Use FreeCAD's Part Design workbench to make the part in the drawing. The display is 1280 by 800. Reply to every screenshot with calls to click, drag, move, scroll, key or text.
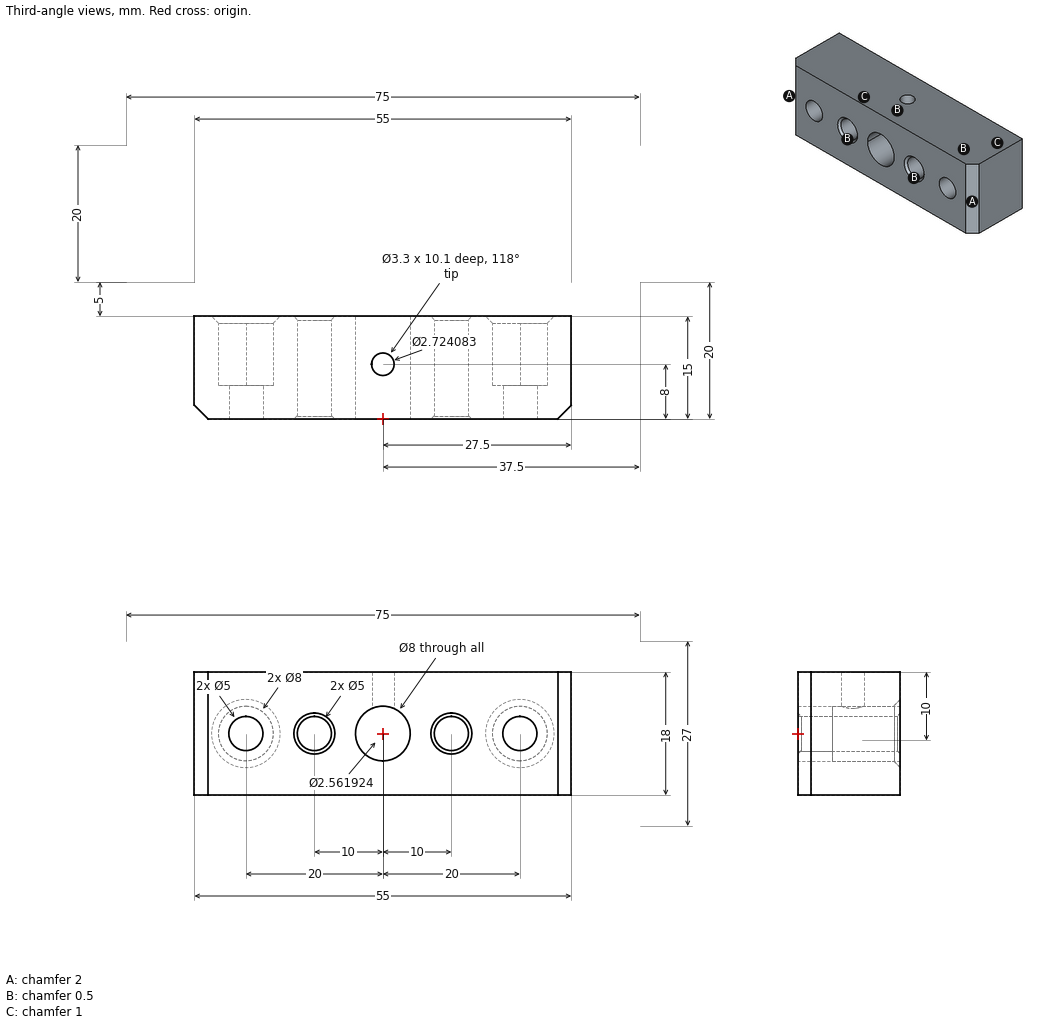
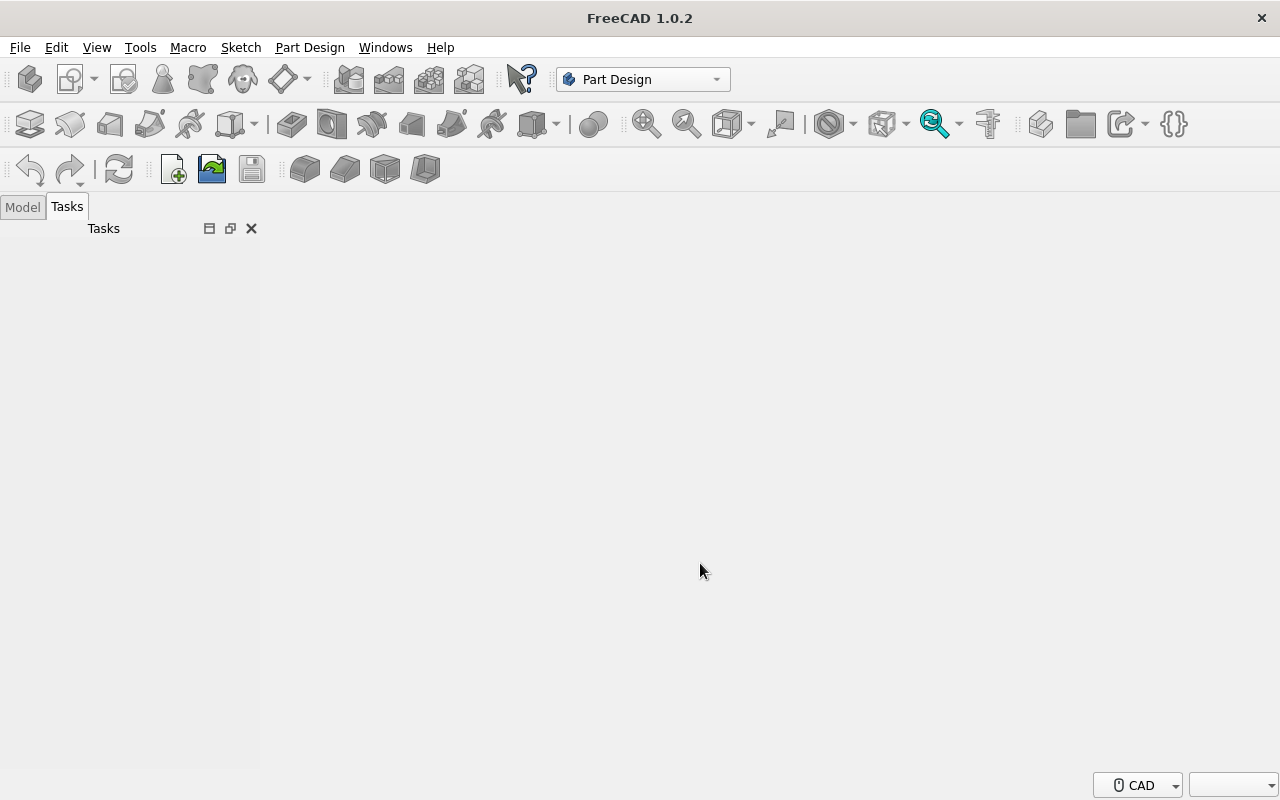
click(172, 170)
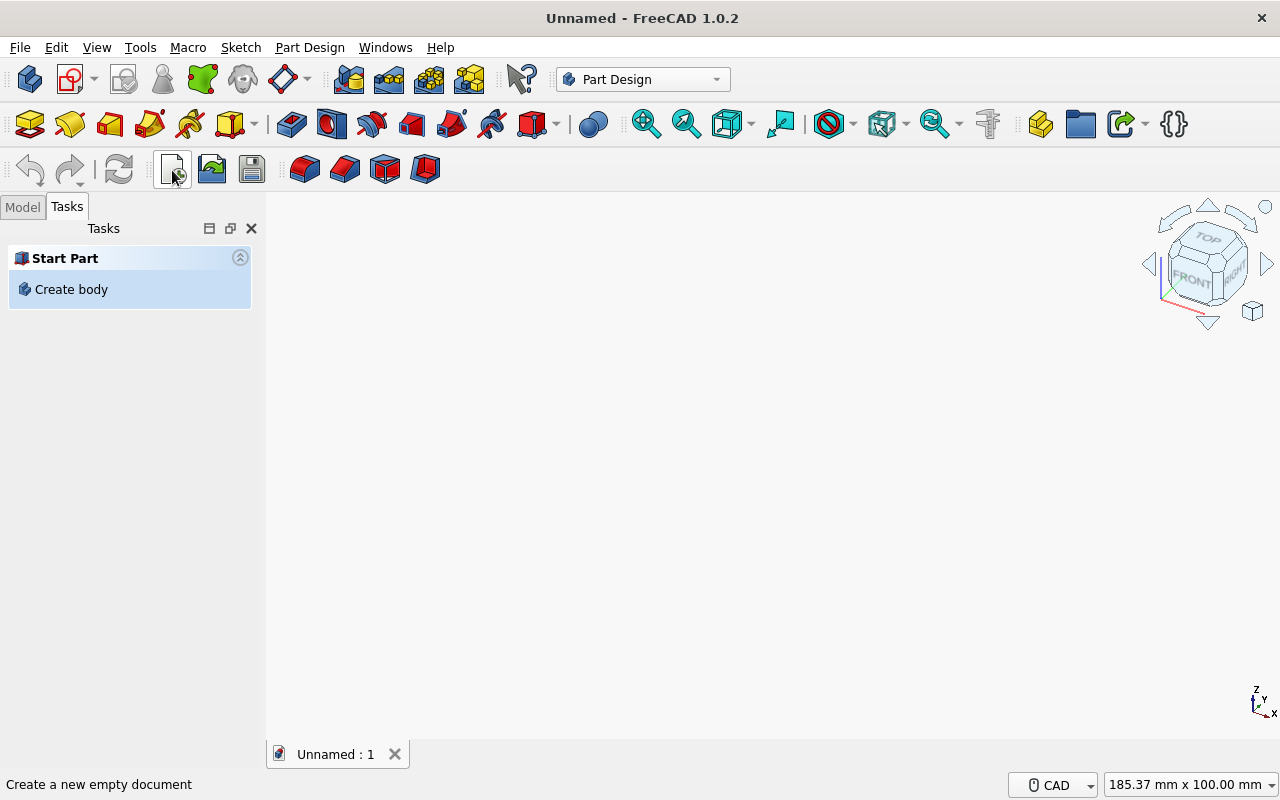
click(70, 80)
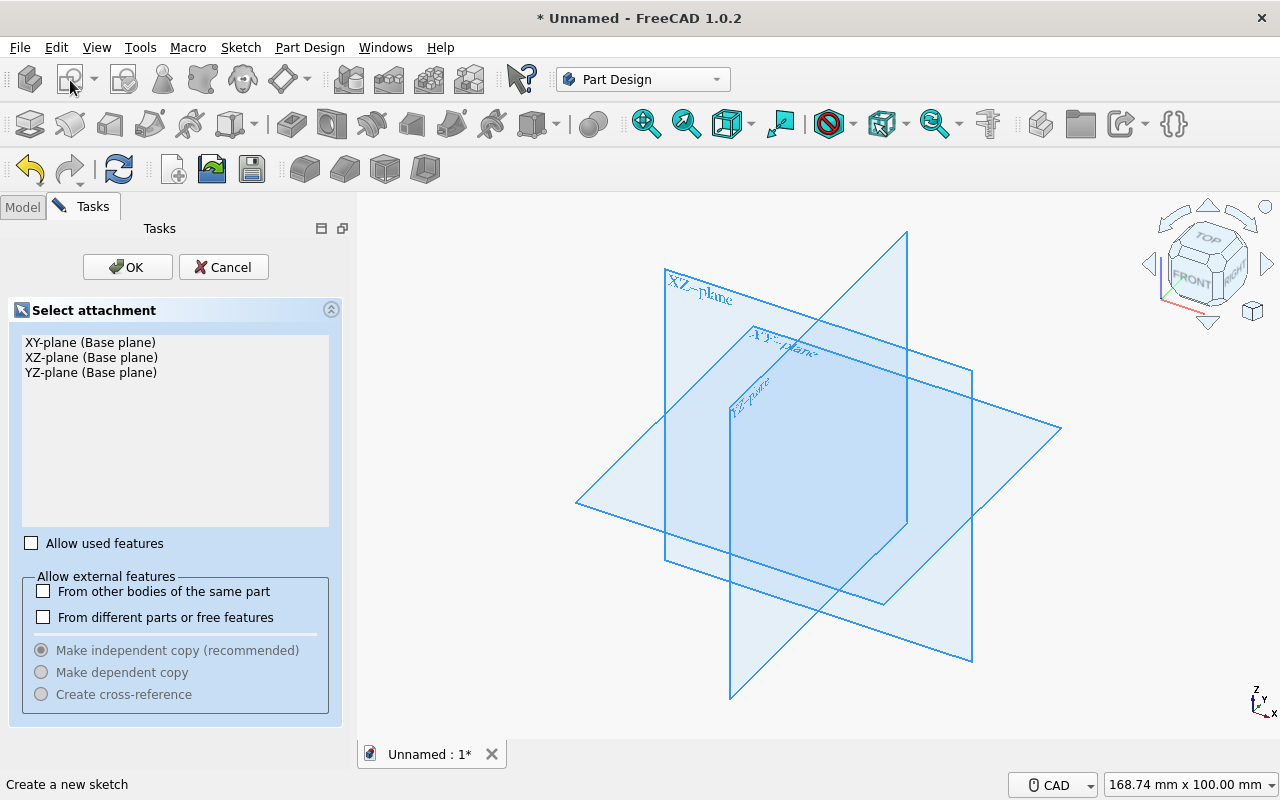
click(82, 358)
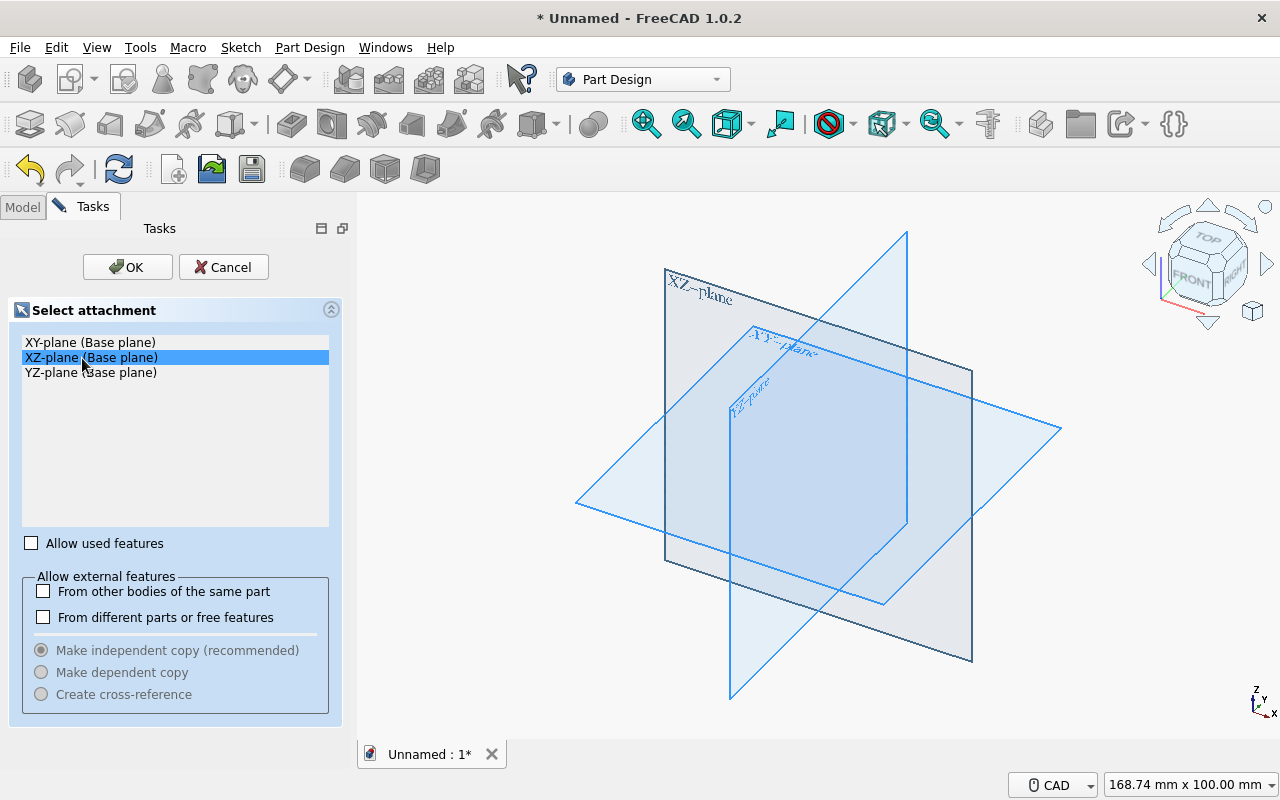
click(128, 267)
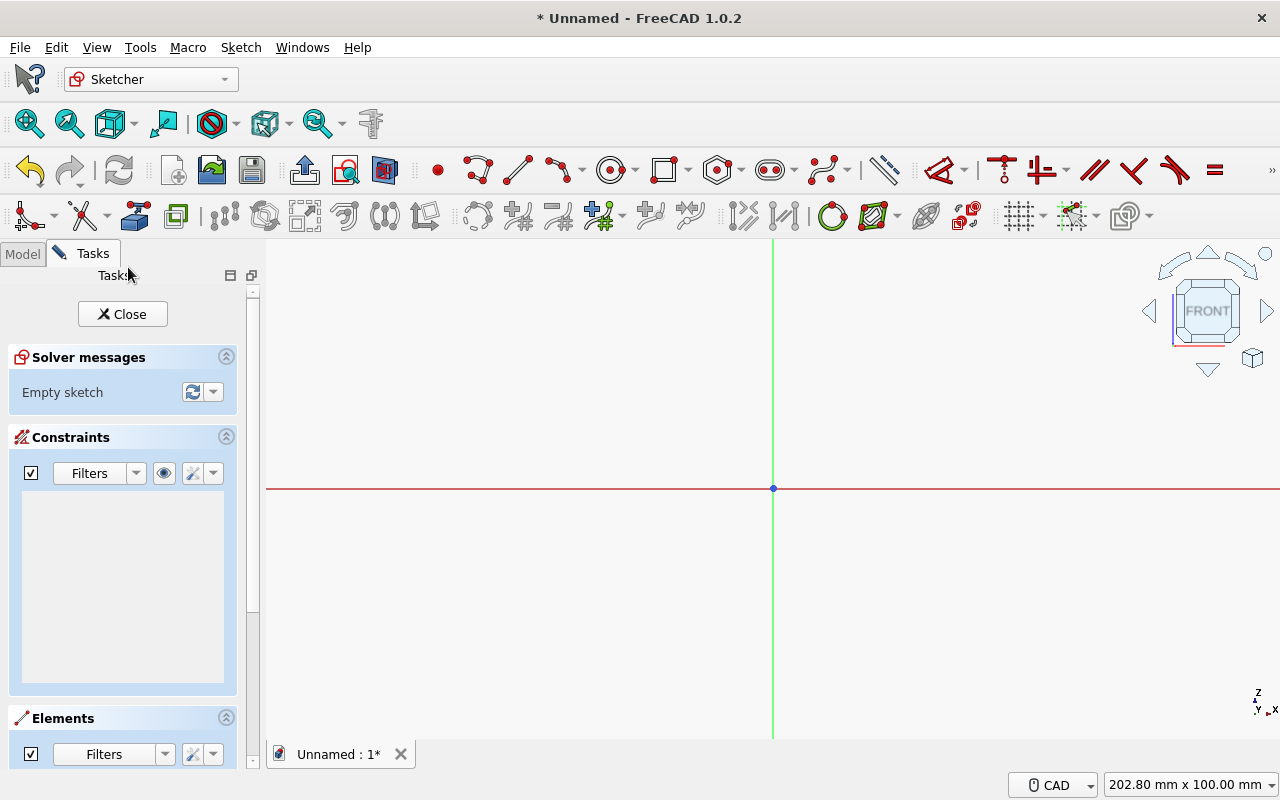
scroll(829, 489, up, 4)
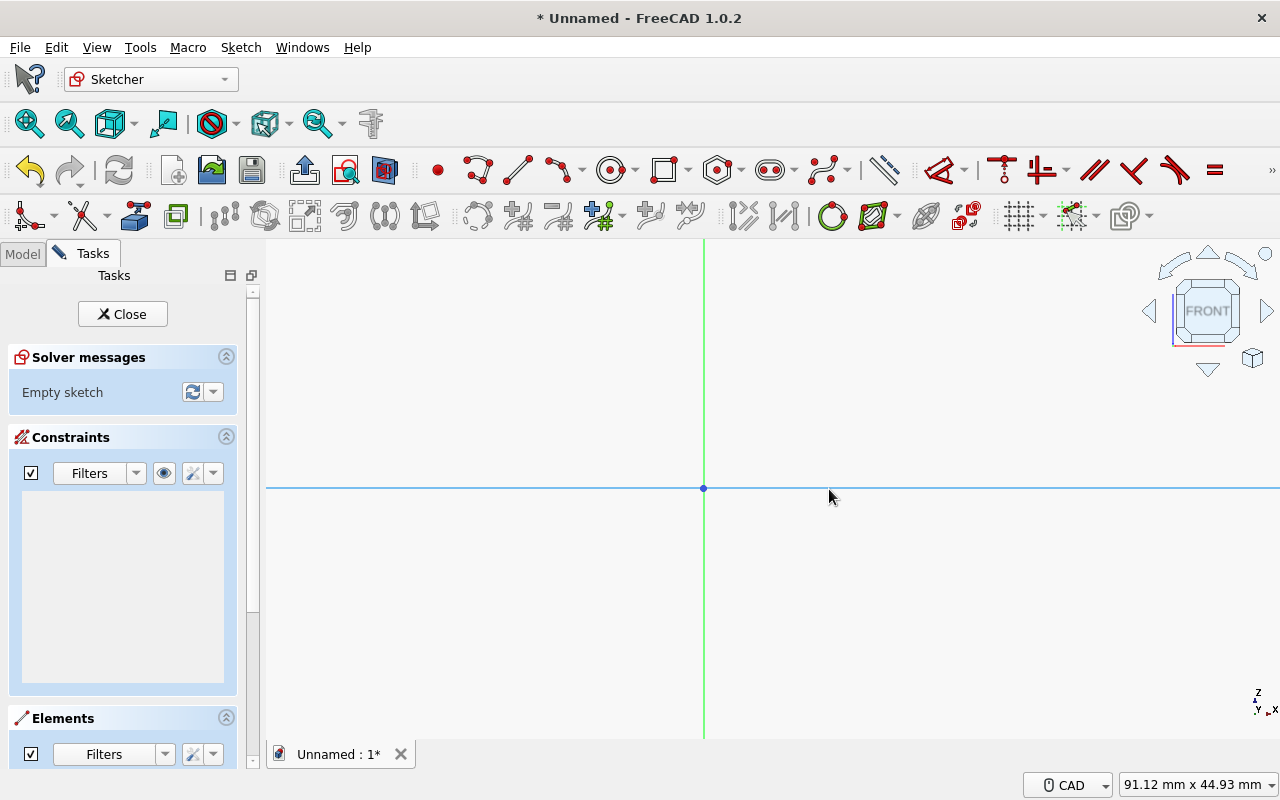
key(g)
key(v)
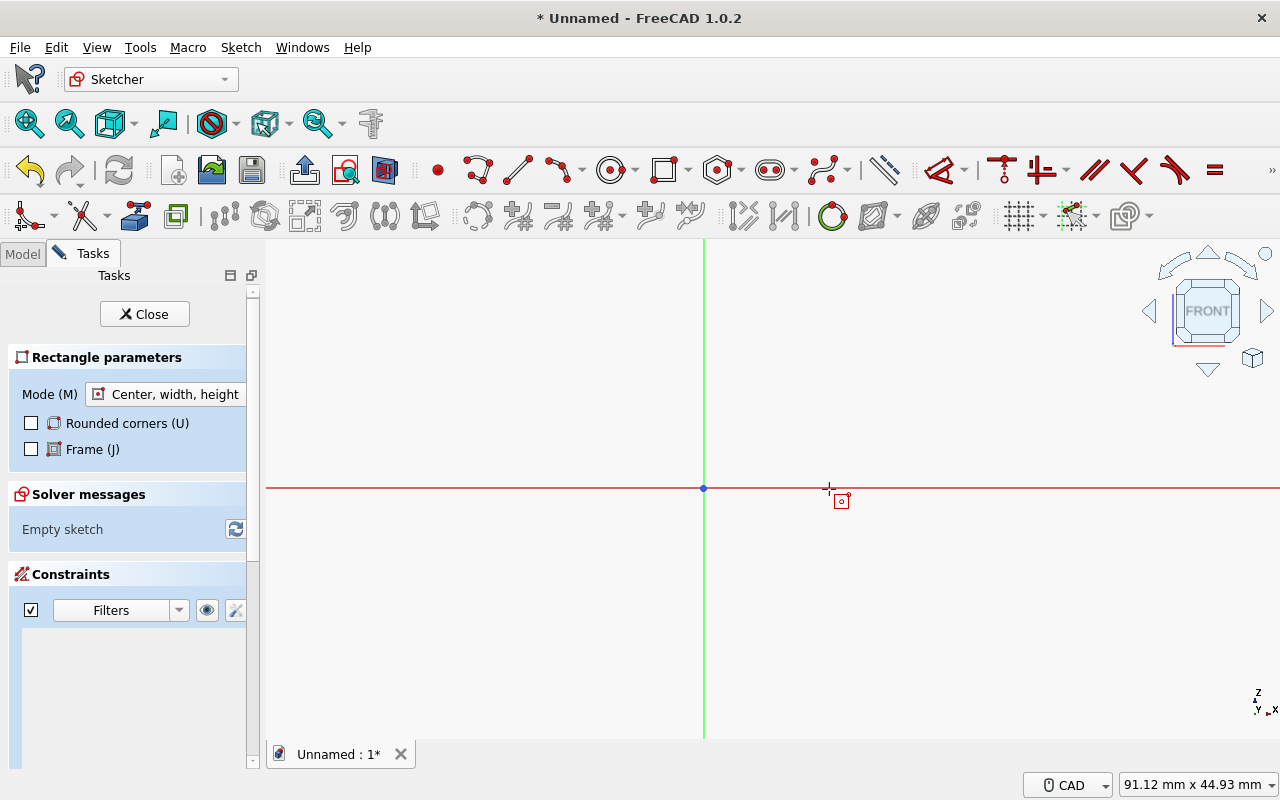
click(704, 488)
move(1010, 388)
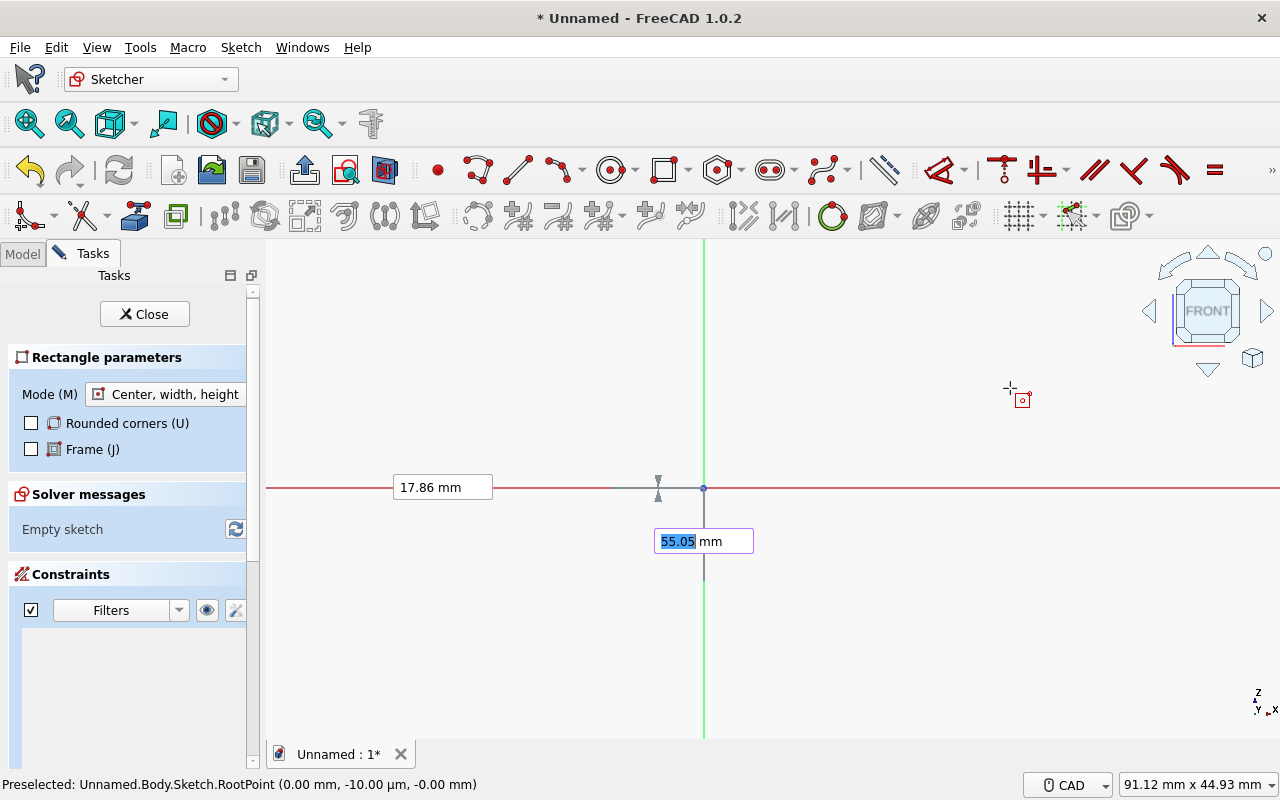
text(55)
key(Tab)
text(18)
key(Return)
key(Escape)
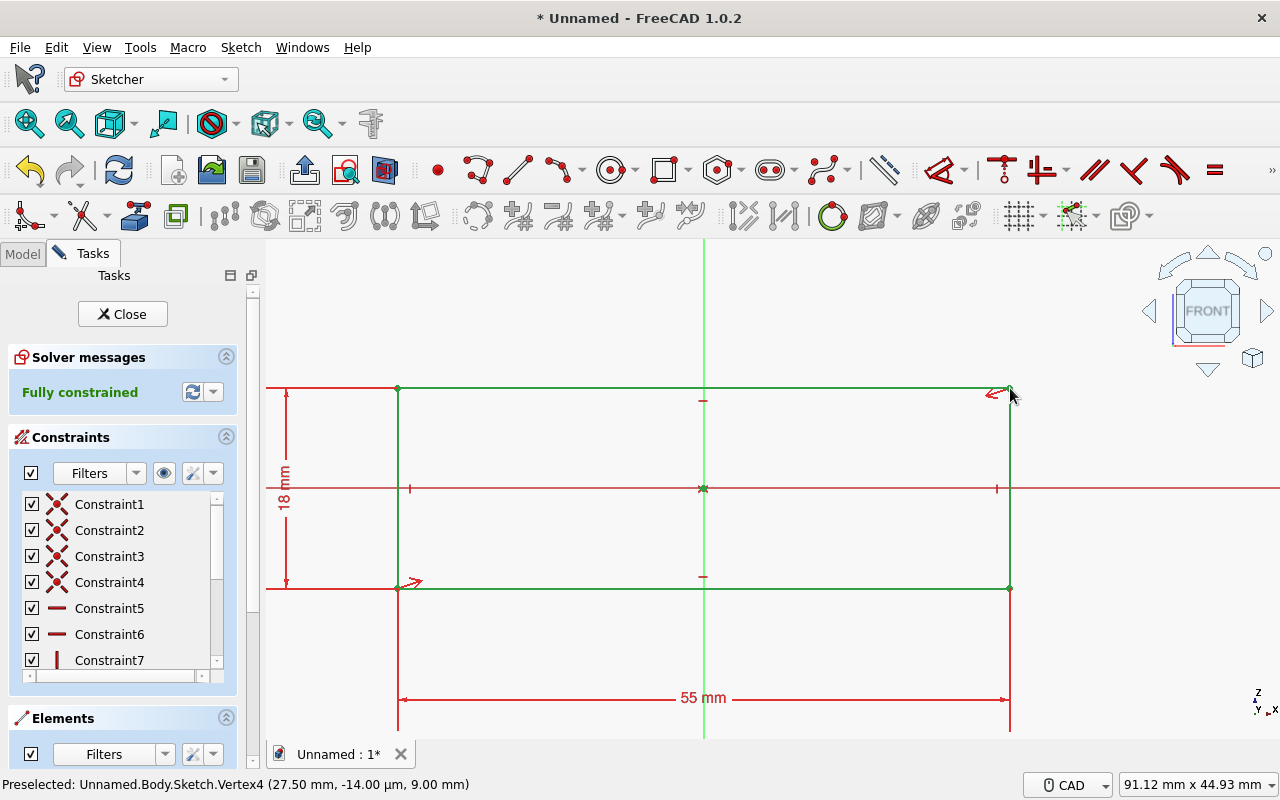
click(123, 314)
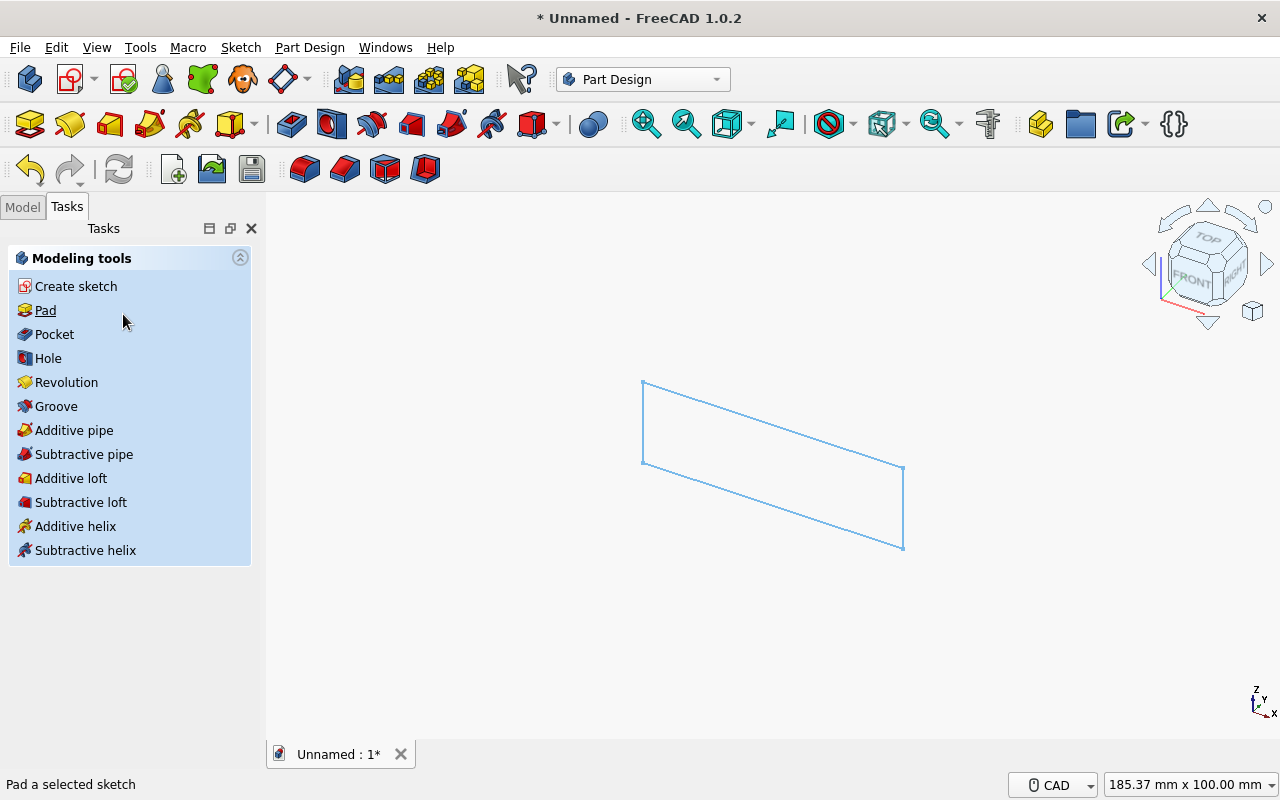
click(30, 124)